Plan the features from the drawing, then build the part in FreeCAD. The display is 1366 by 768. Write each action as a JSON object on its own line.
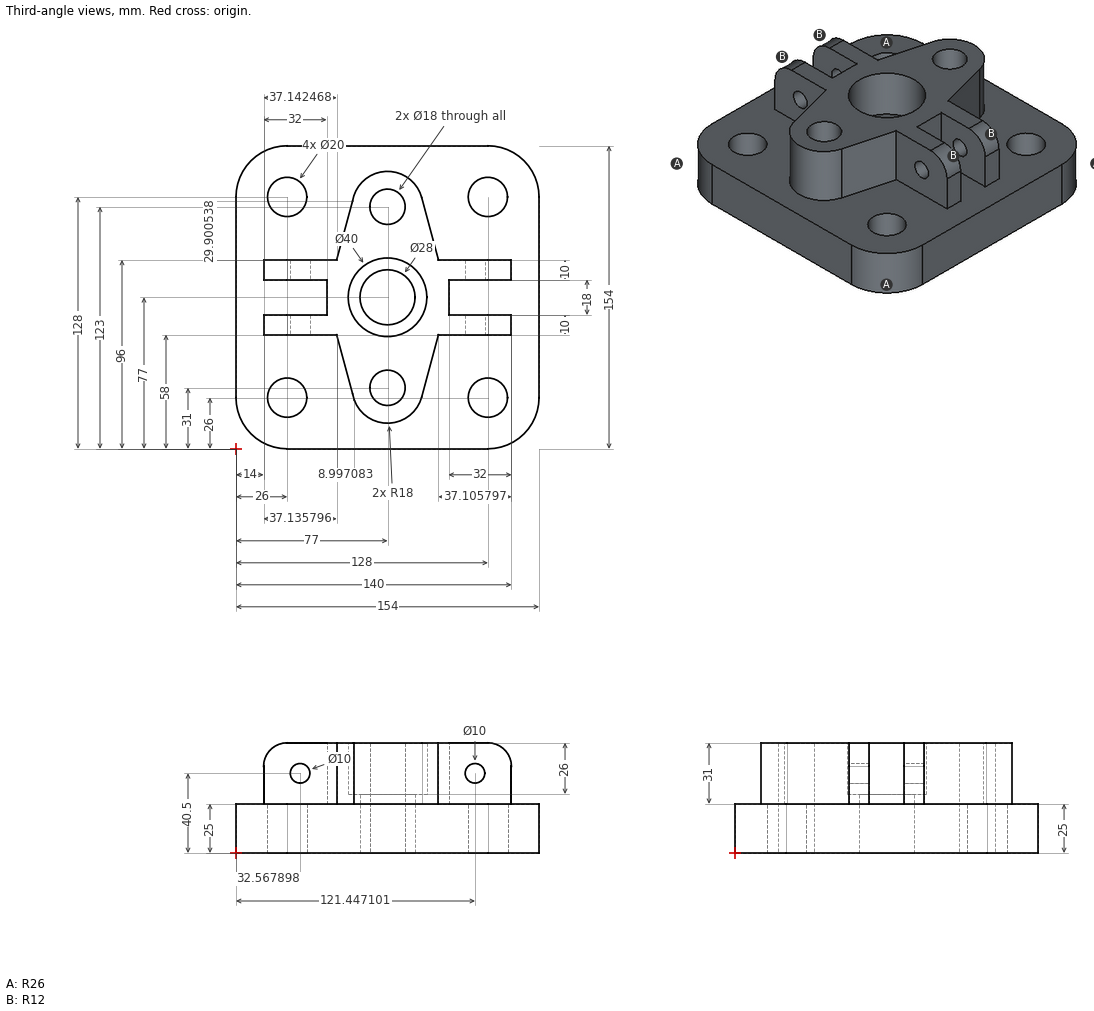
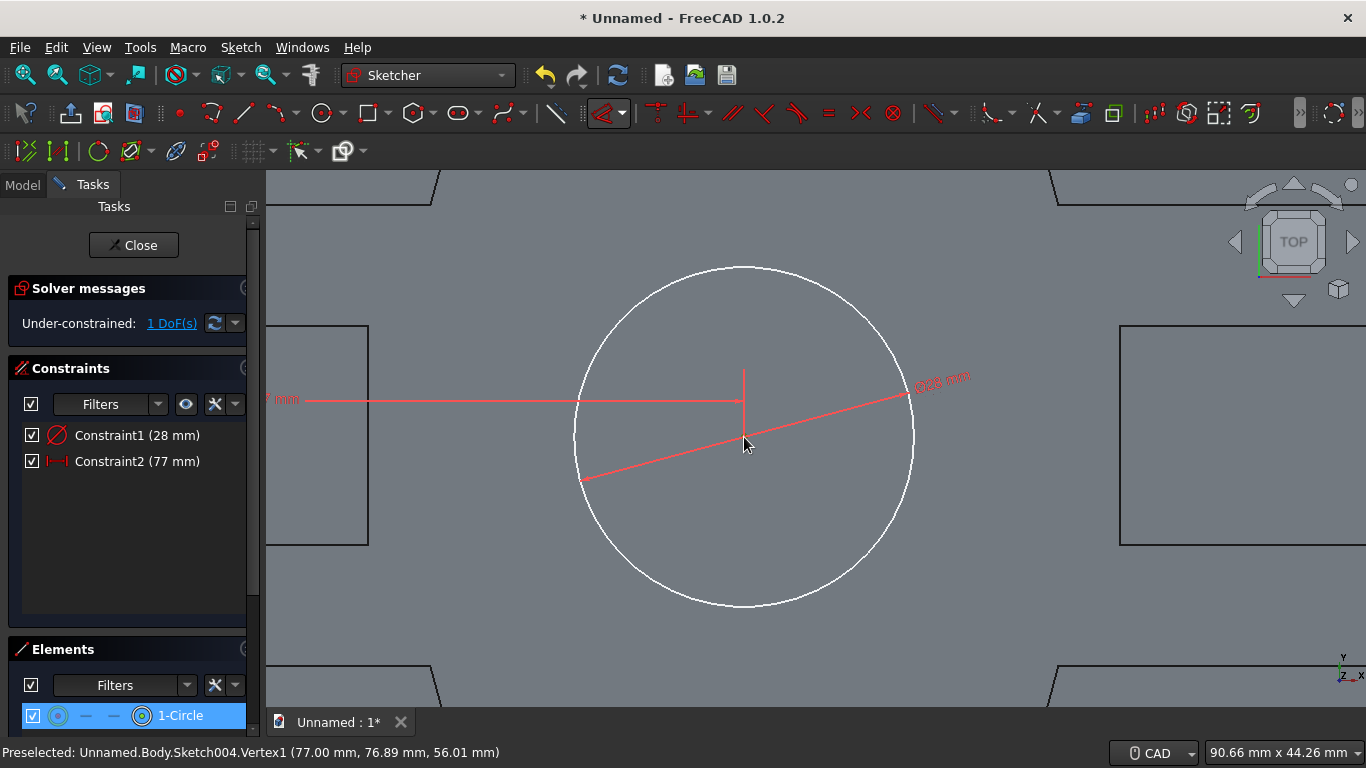
{"action": "left_click", "coordinate": [624, 114]}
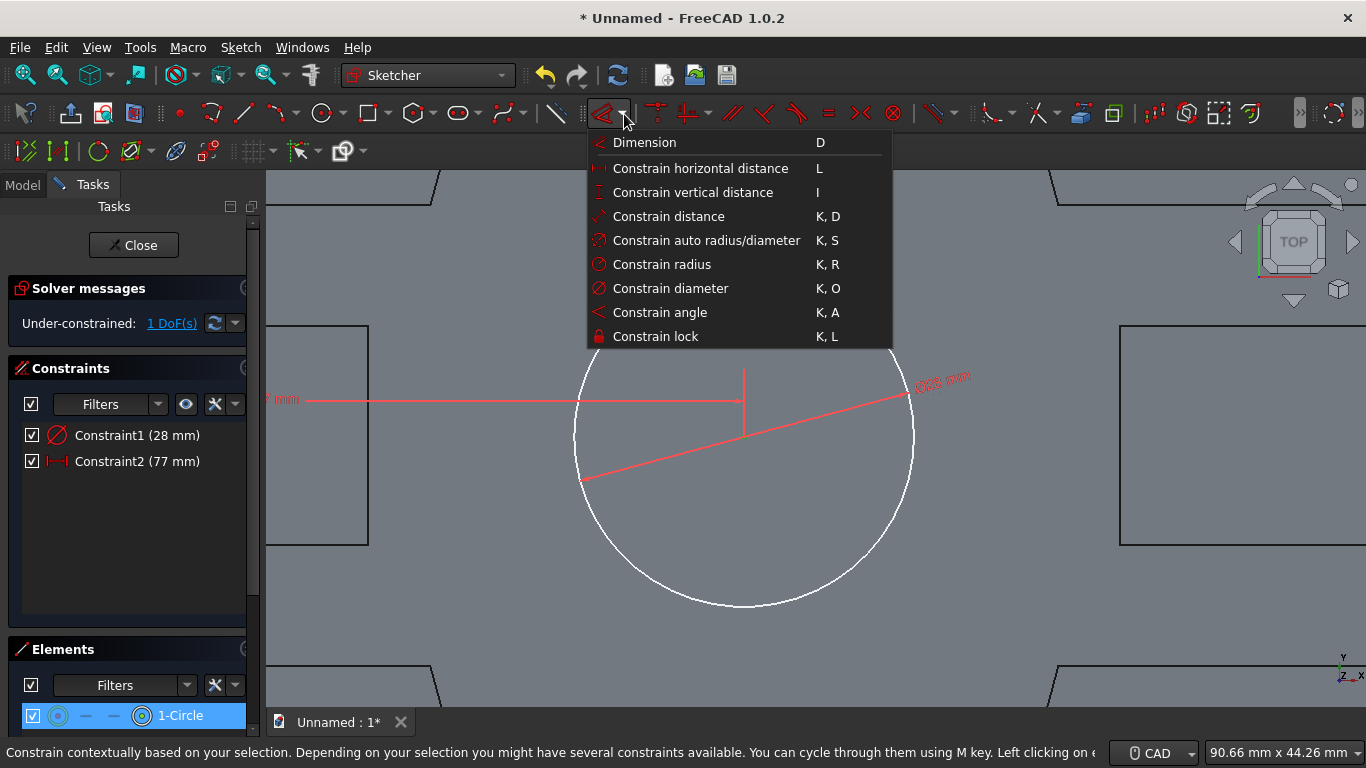
{"action": "left_click", "coordinate": [740, 192]}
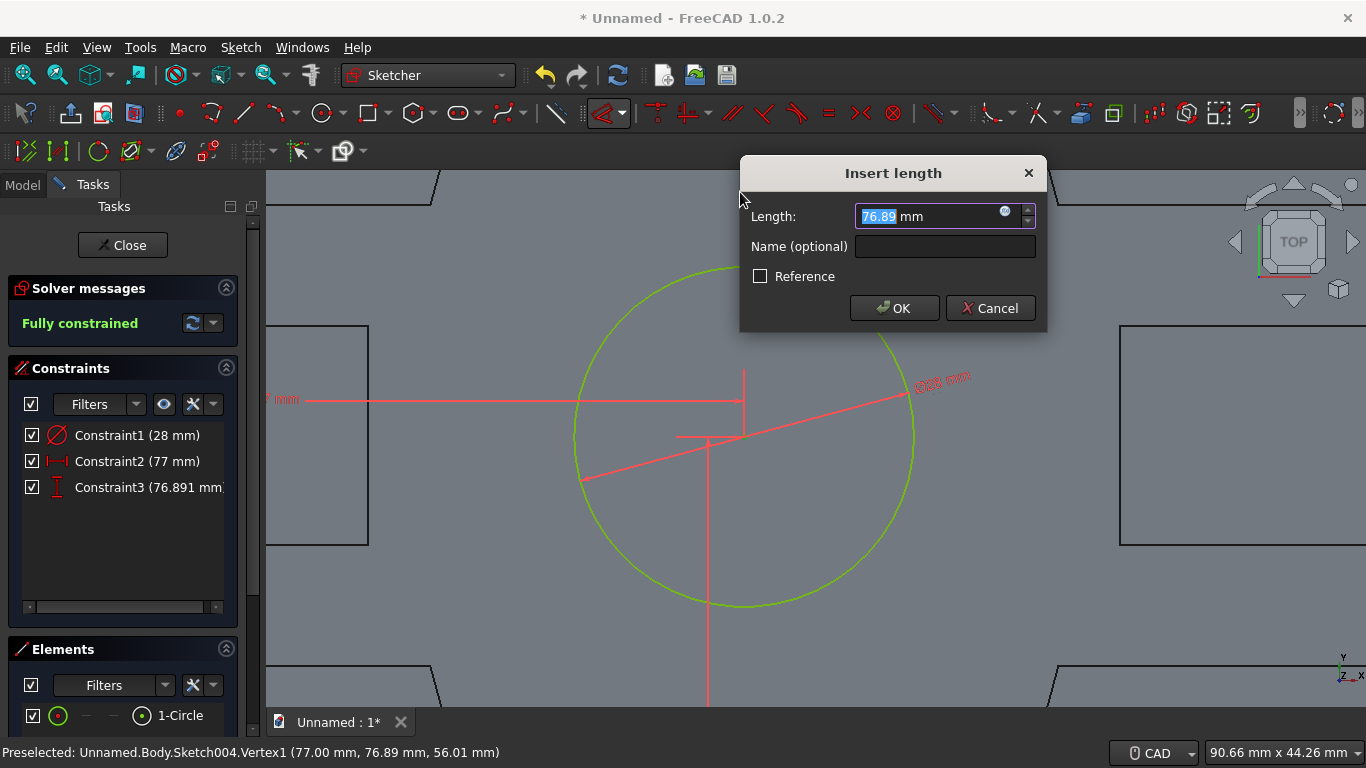
{"action": "type", "text": "77"}
{"action": "key", "text": "Return"}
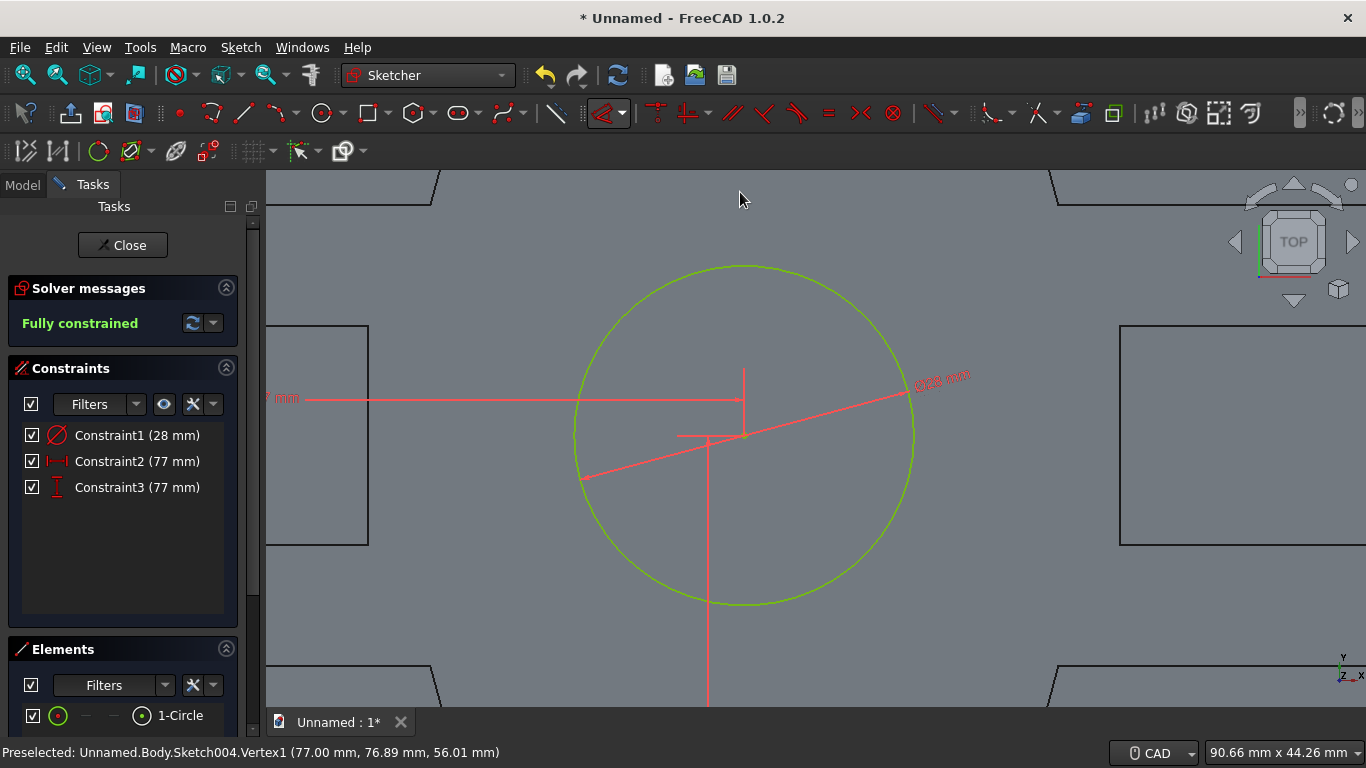
{"action": "left_click", "coordinate": [123, 245]}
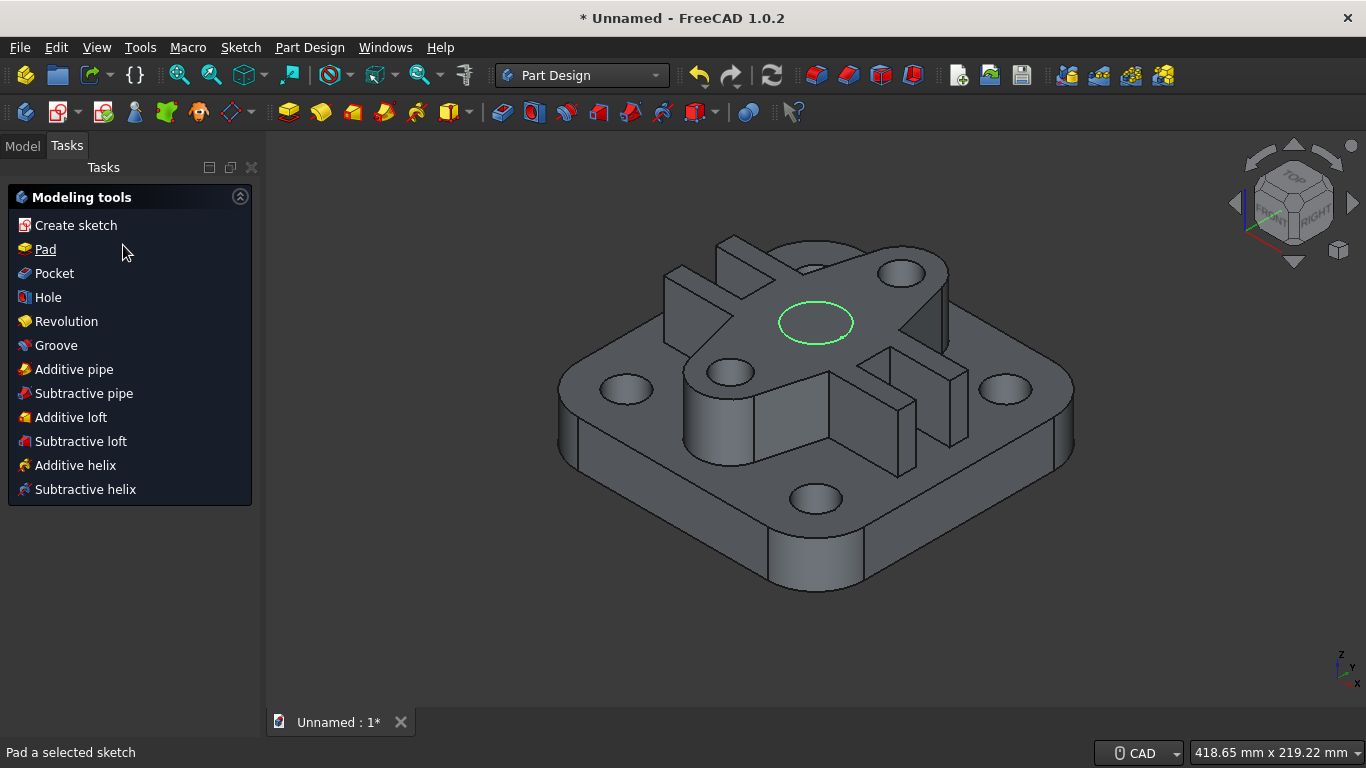
{"action": "left_click", "coordinate": [504, 112]}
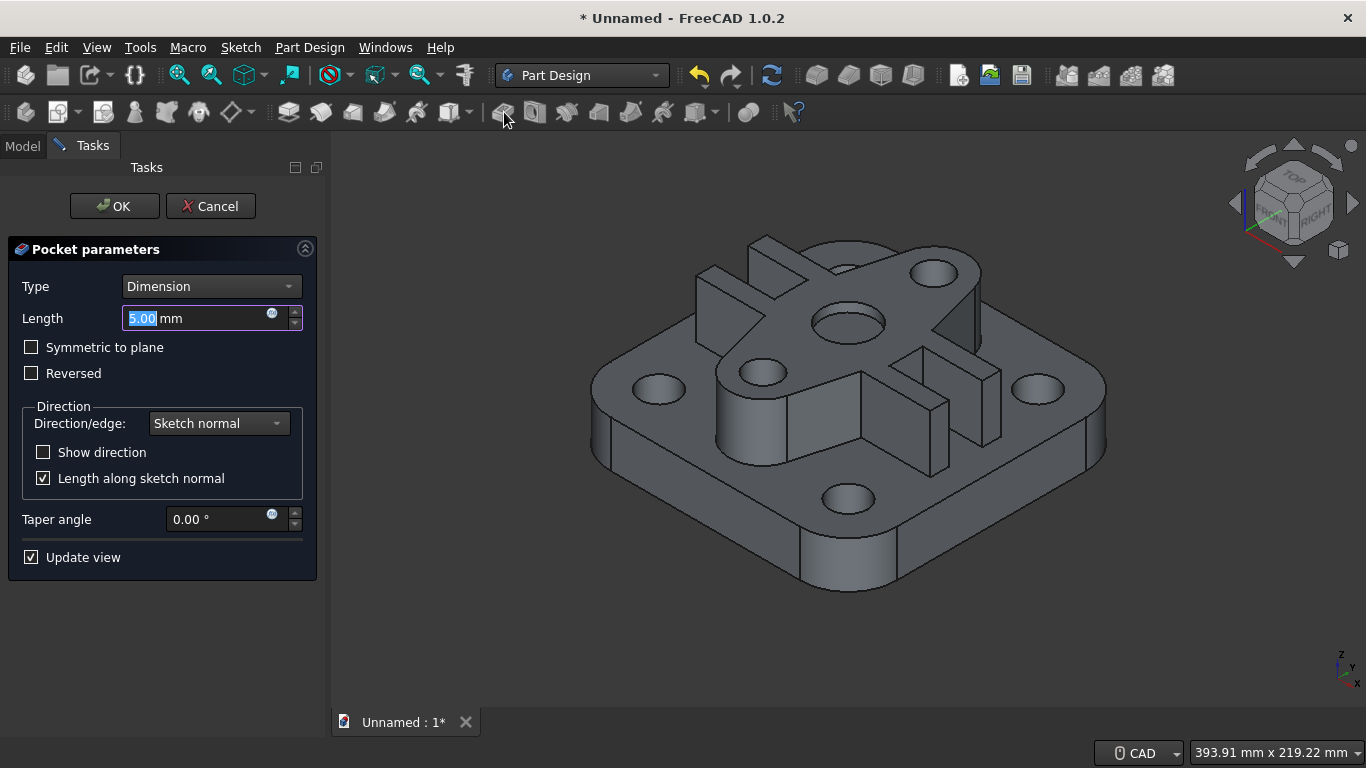
{"action": "left_click", "coordinate": [212, 286]}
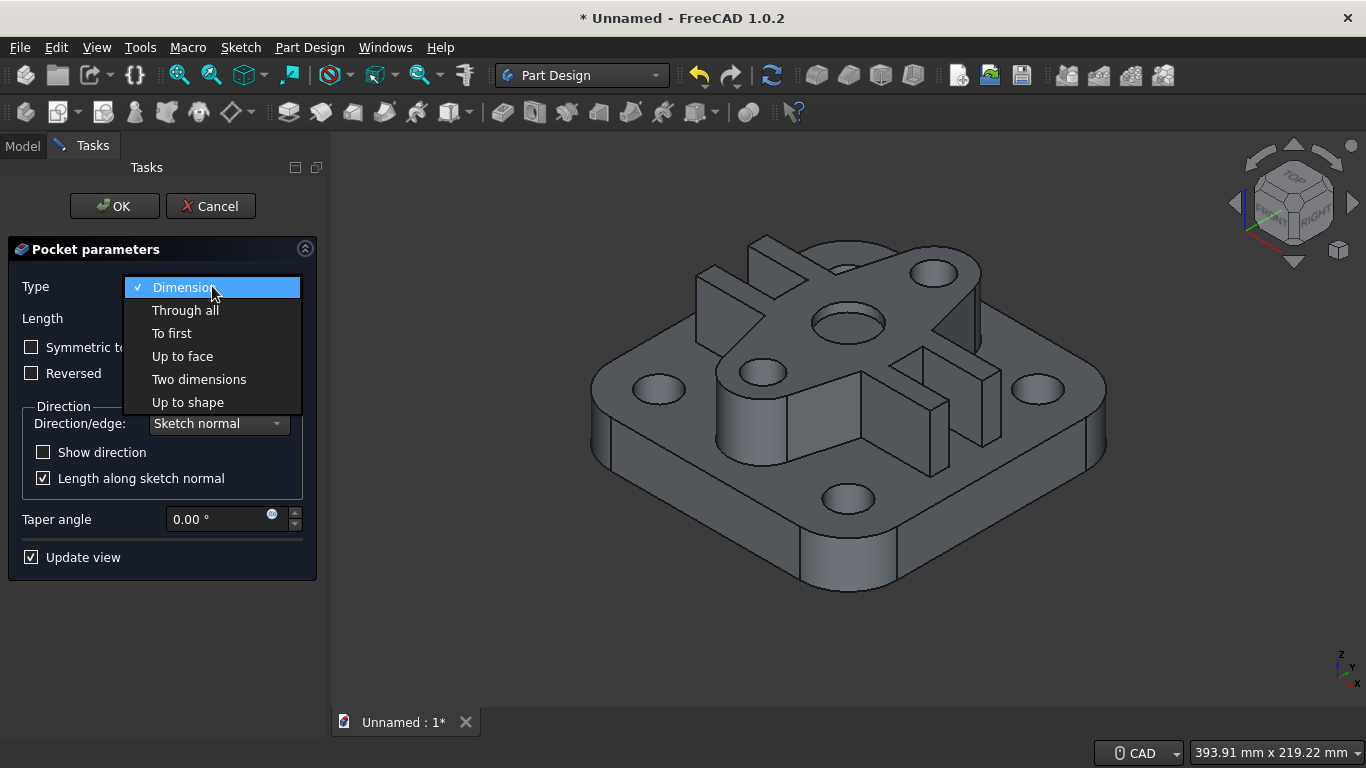
{"action": "left_click", "coordinate": [212, 310]}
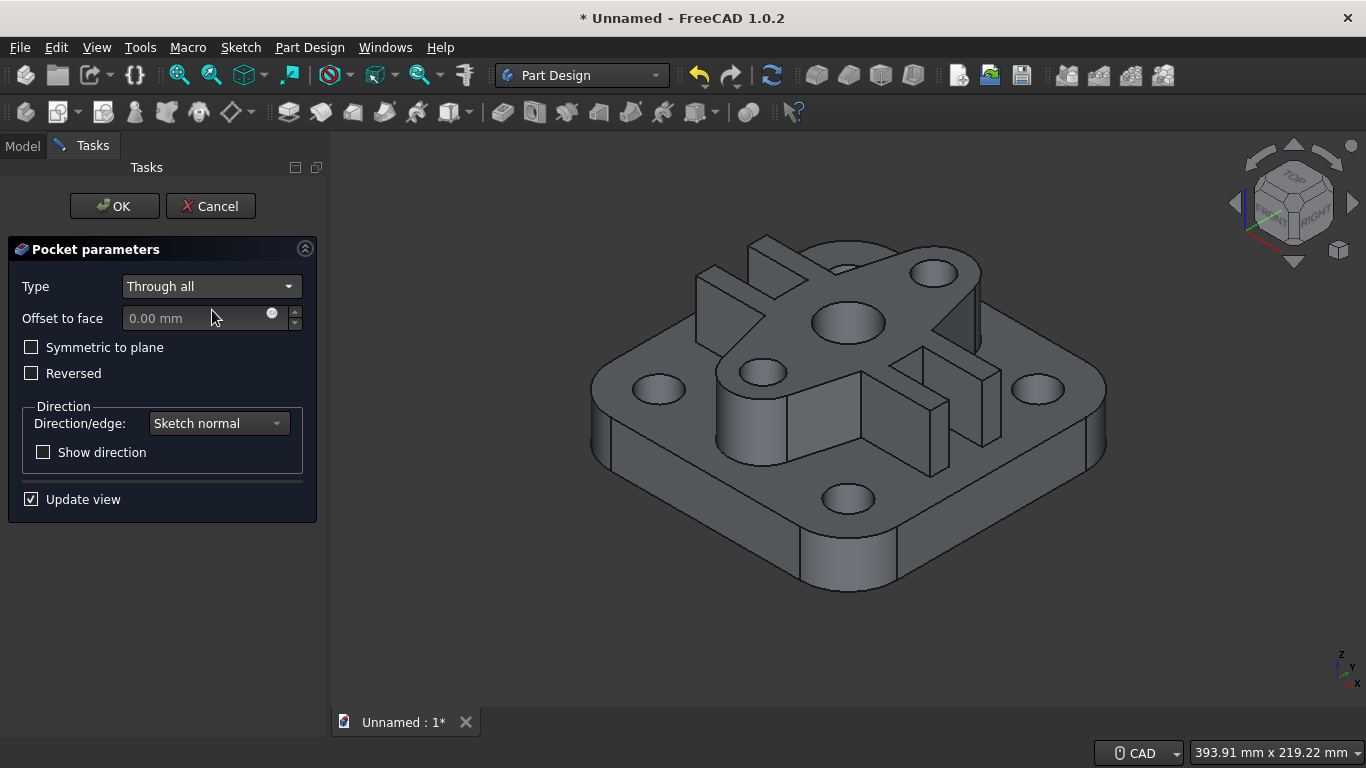
{"action": "left_click", "coordinate": [115, 206]}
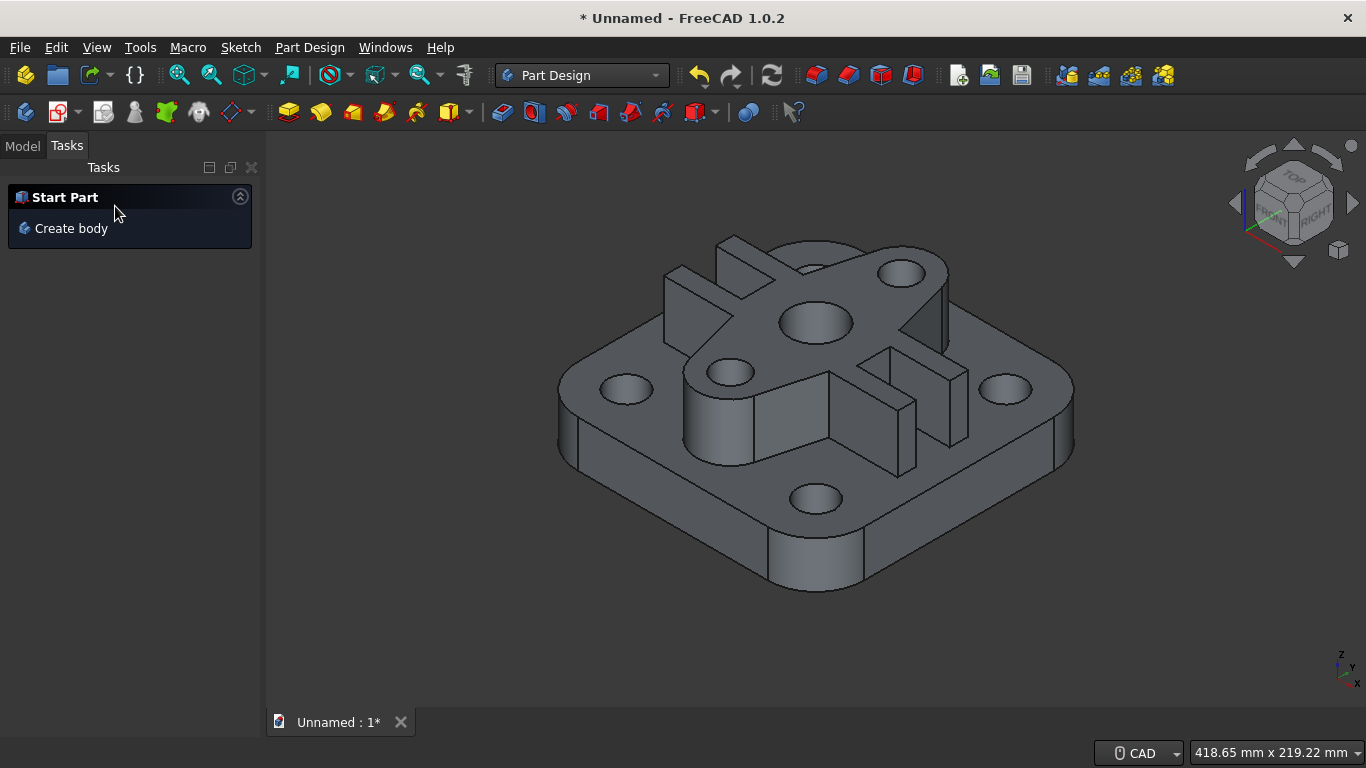
{"action": "left_click", "coordinate": [883, 322]}